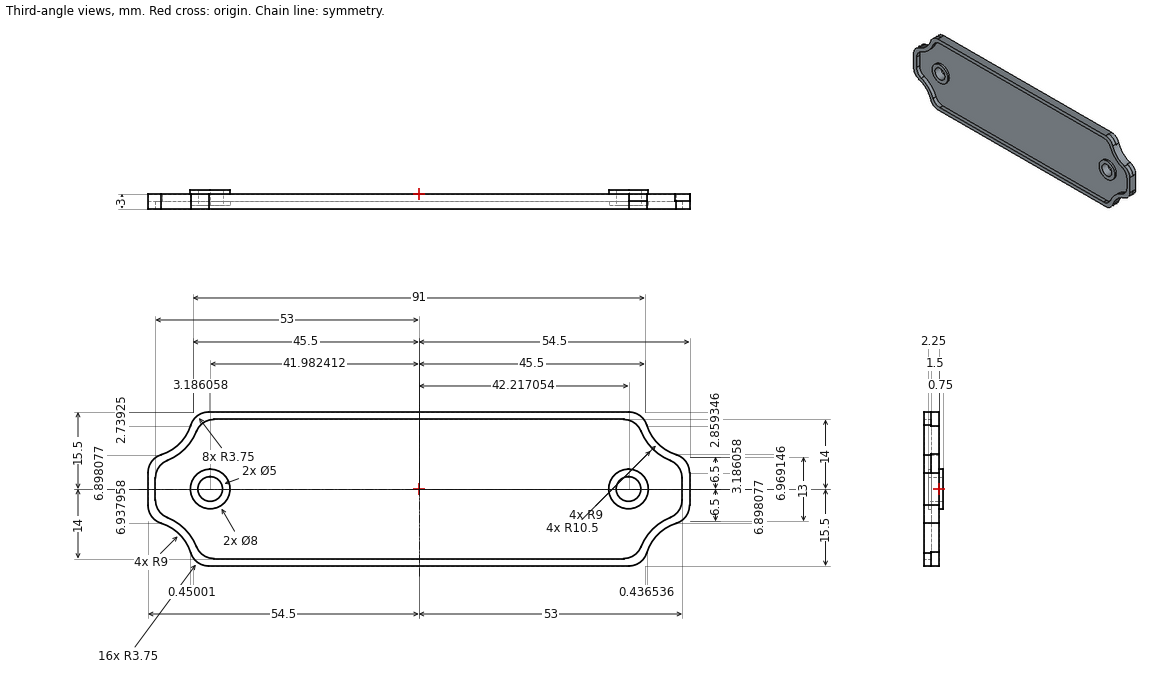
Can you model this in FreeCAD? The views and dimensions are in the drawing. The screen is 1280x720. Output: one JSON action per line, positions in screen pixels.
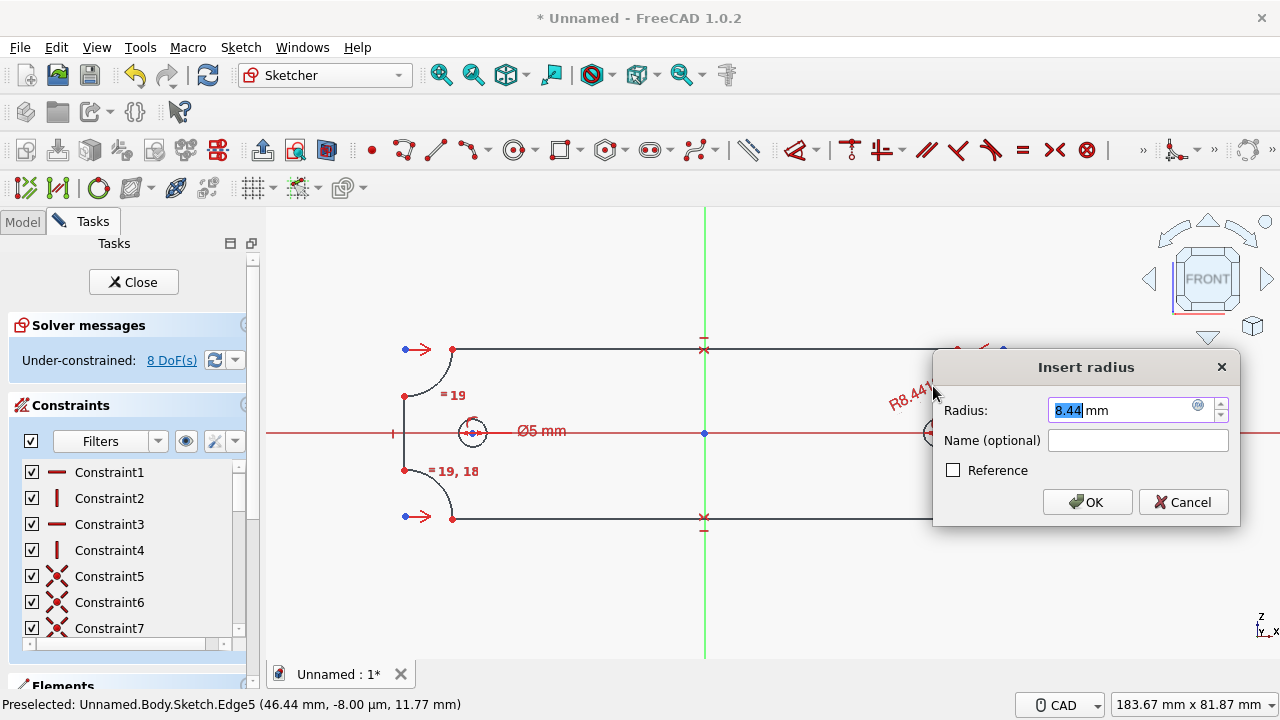
{"action": "type", "text": "9"}
{"action": "key", "text": "Return"}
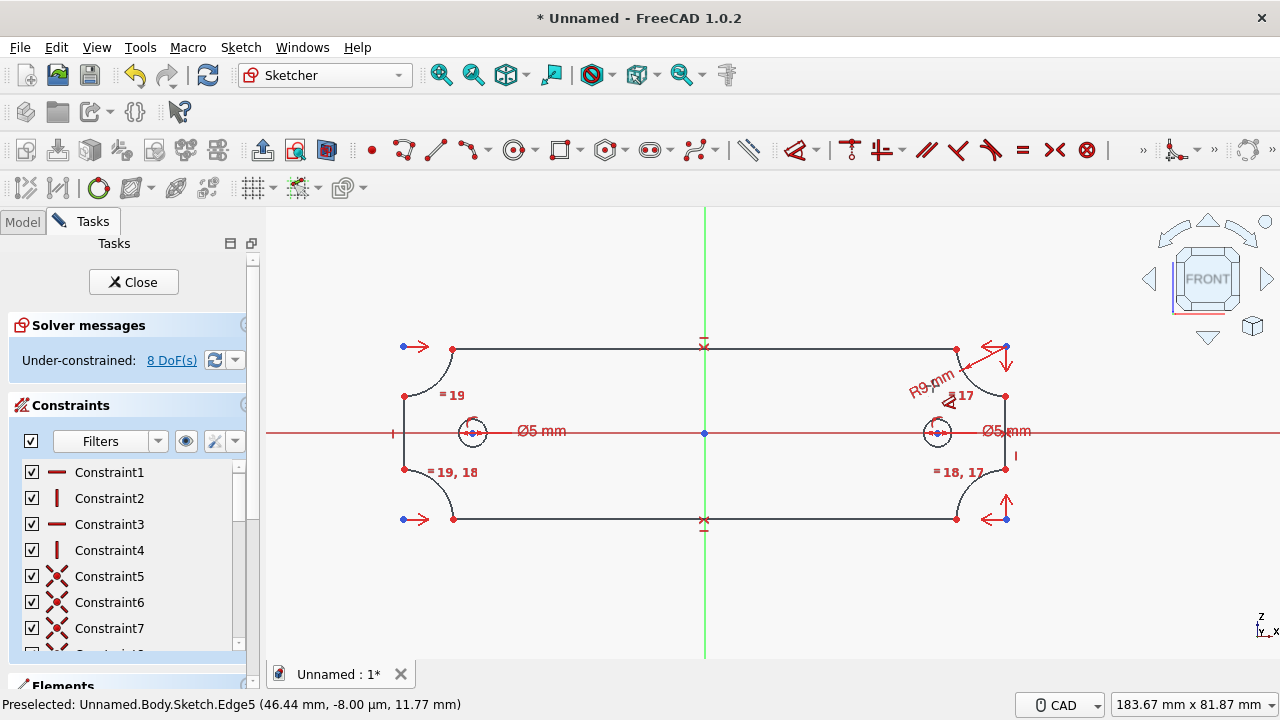
{"action": "left_click", "coordinate": [604, 349]}
{"action": "left_click", "coordinate": [589, 315]}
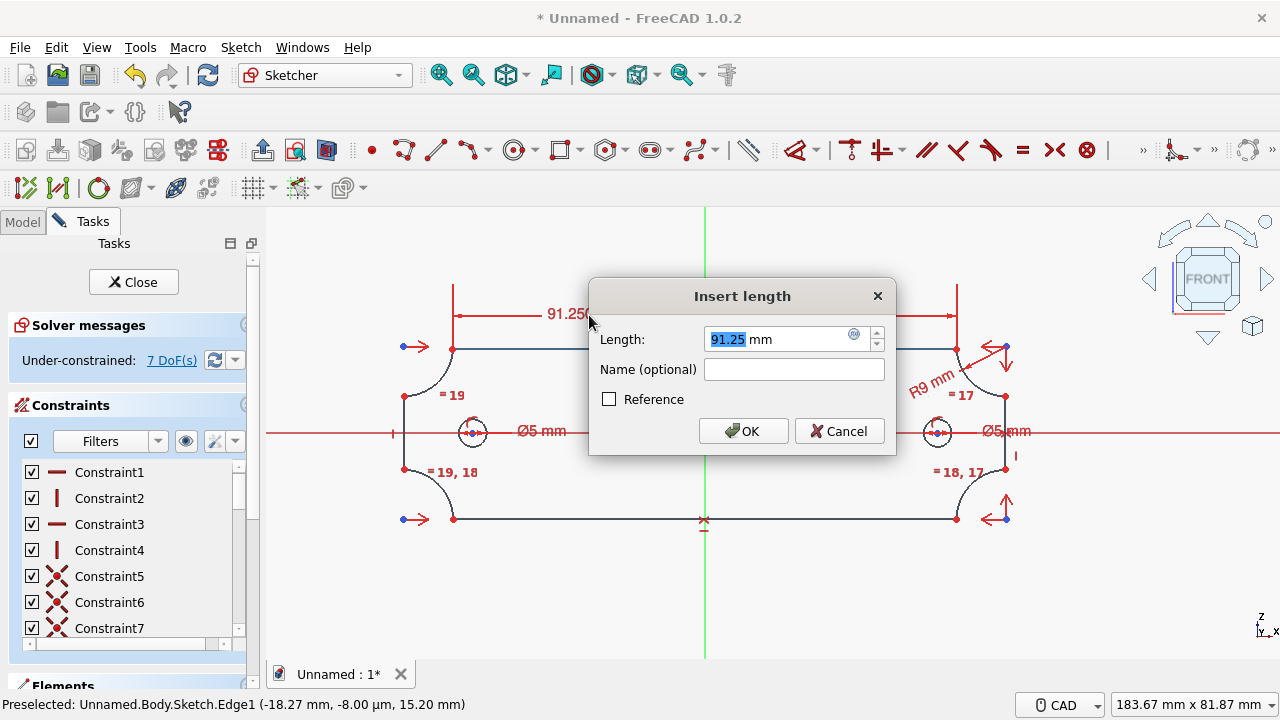
{"action": "type", "text": "91"}
{"action": "key", "text": "Return"}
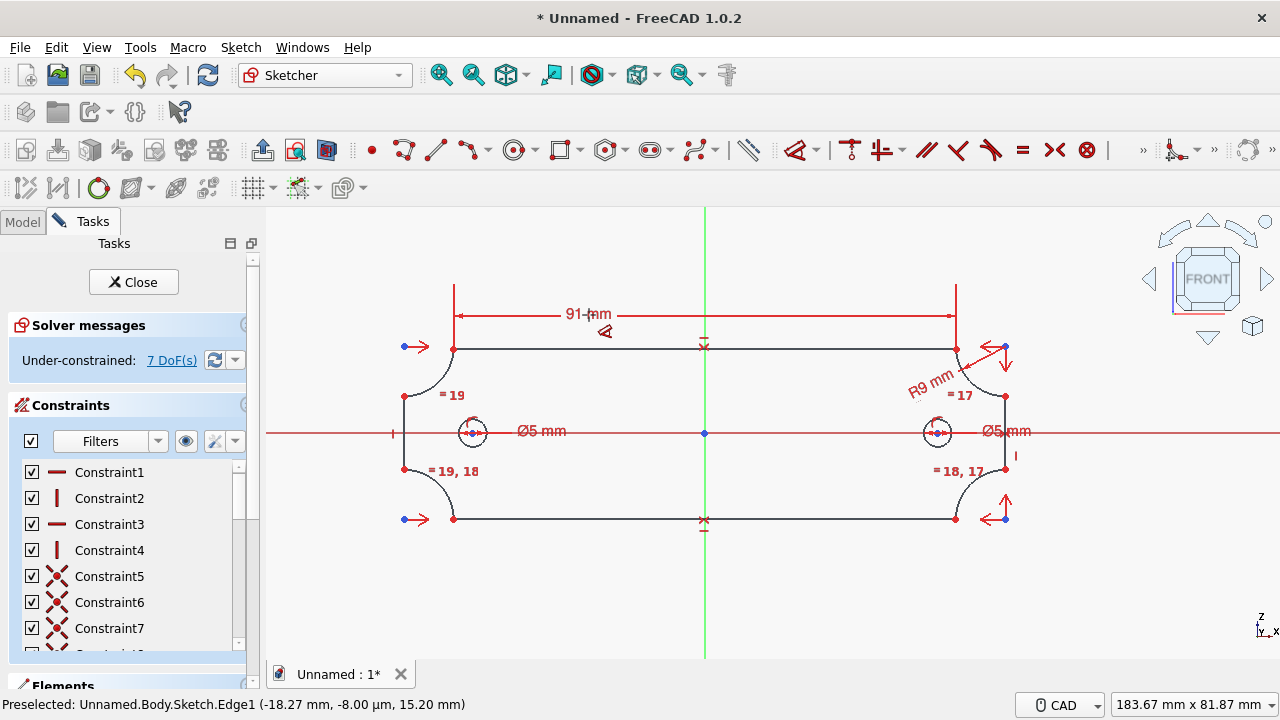
{"action": "left_click", "coordinate": [1005, 418]}
{"action": "left_click", "coordinate": [1039, 416]}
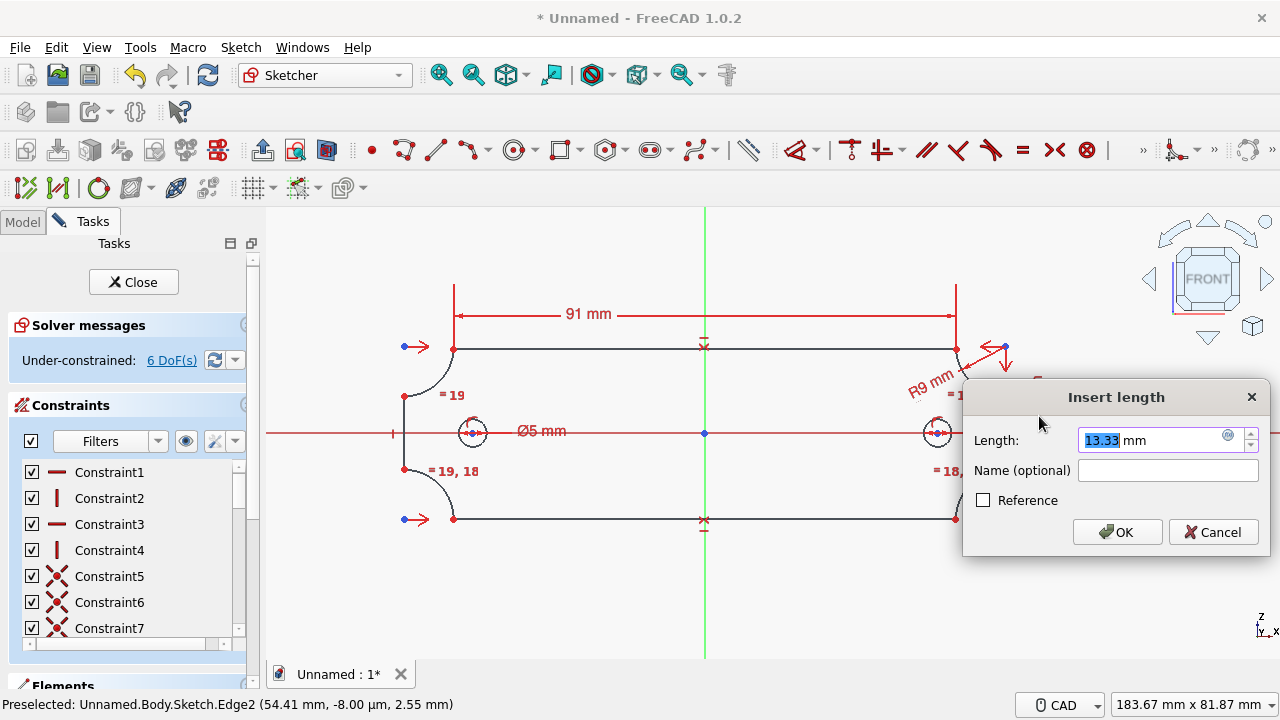
{"action": "type", "text": "13"}
{"action": "key", "text": "Return"}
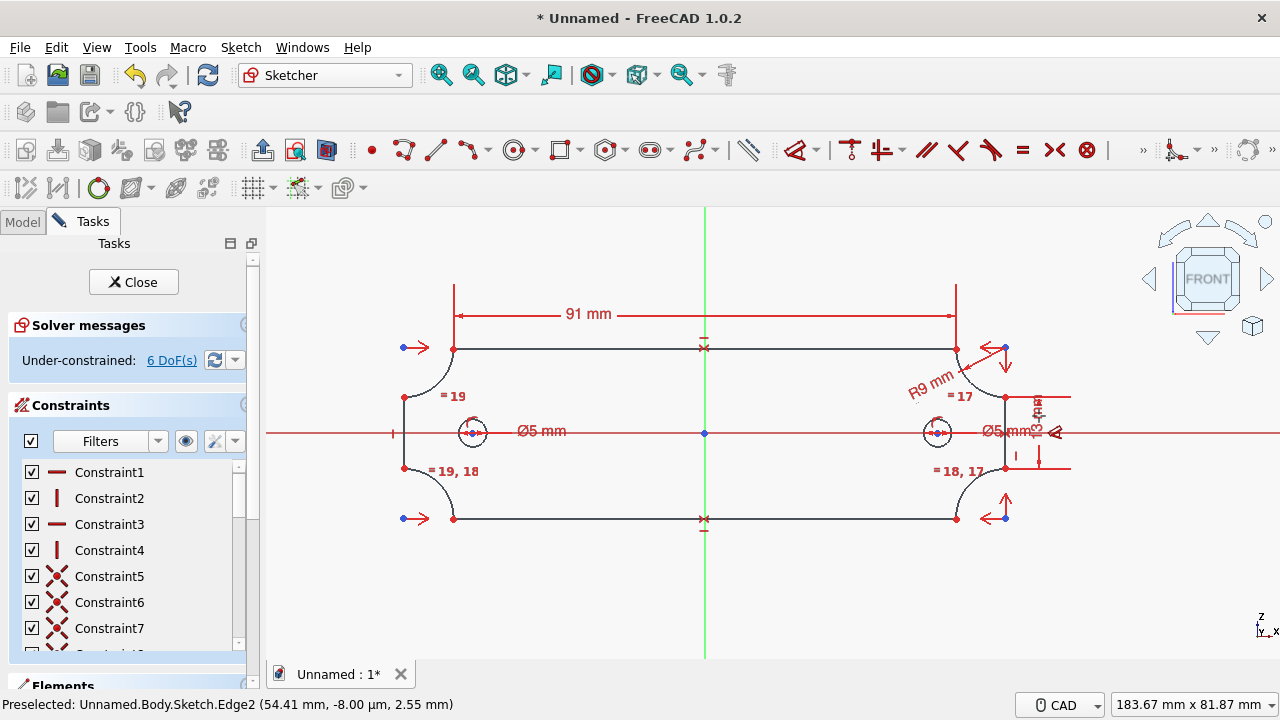
{"action": "left_click", "coordinate": [454, 349]}
{"action": "left_click", "coordinate": [420, 372]}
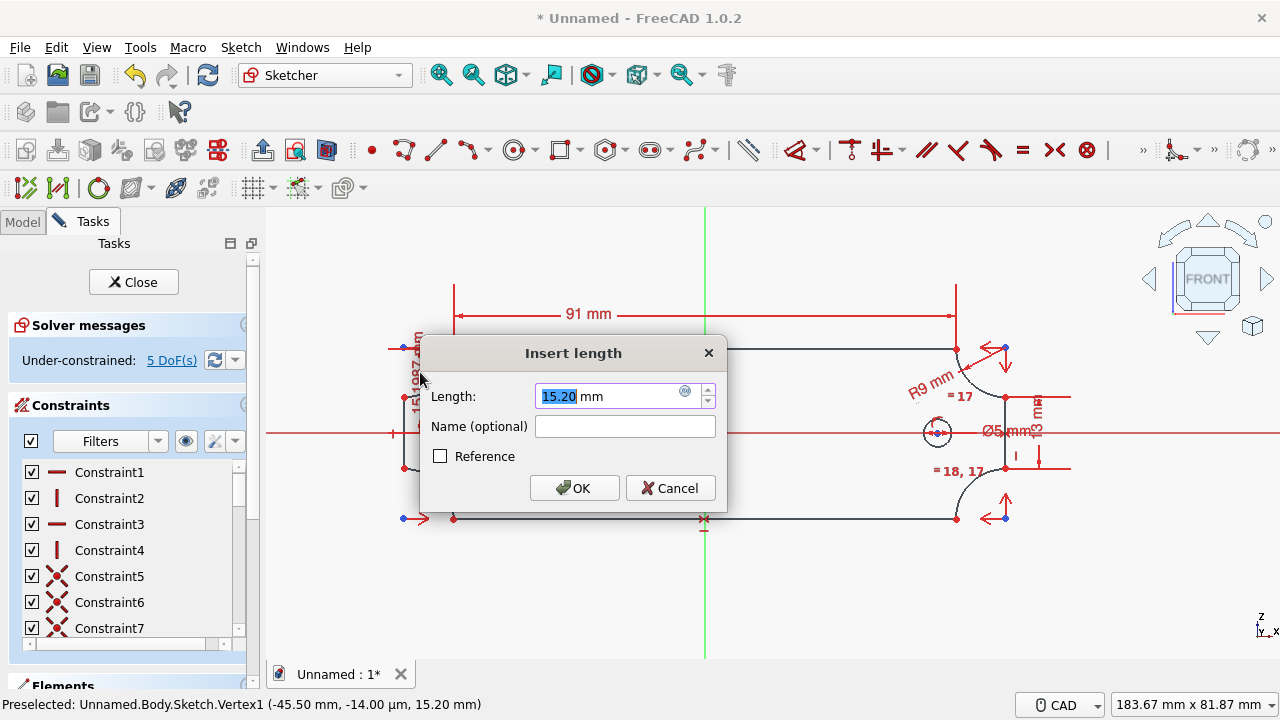
{"action": "type", "text": "15.5"}
{"action": "key", "text": "Return"}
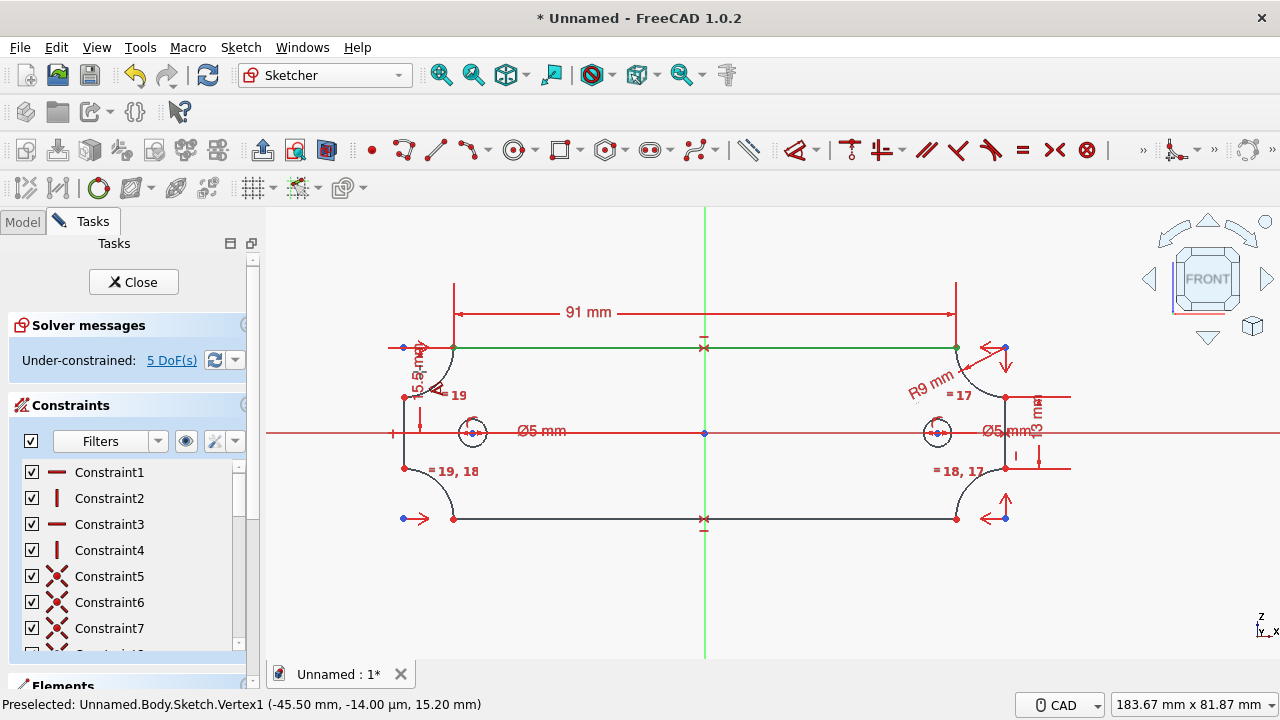
{"action": "left_click", "coordinate": [1005, 397]}
{"action": "left_click", "coordinate": [855, 363]}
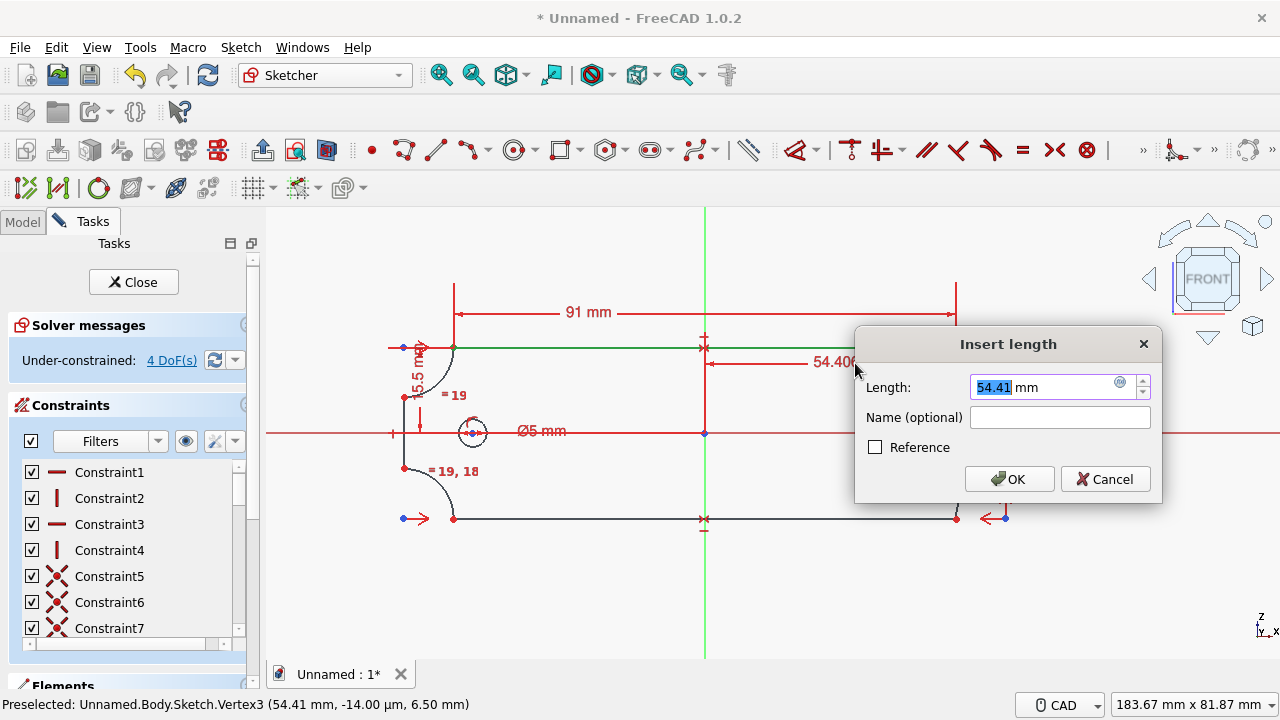
{"action": "type", "text": "54.5"}
{"action": "key", "text": "Return"}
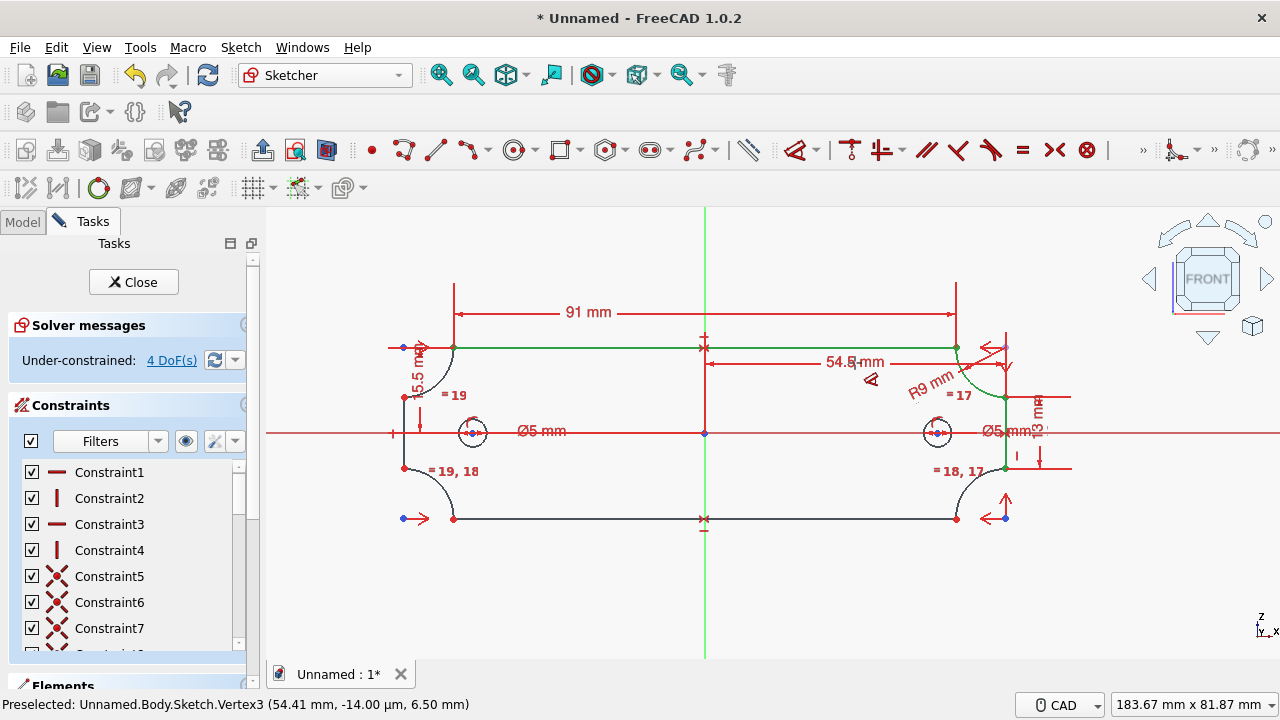
{"action": "left_click", "coordinate": [956, 519]}
{"action": "left_click", "coordinate": [990, 456]}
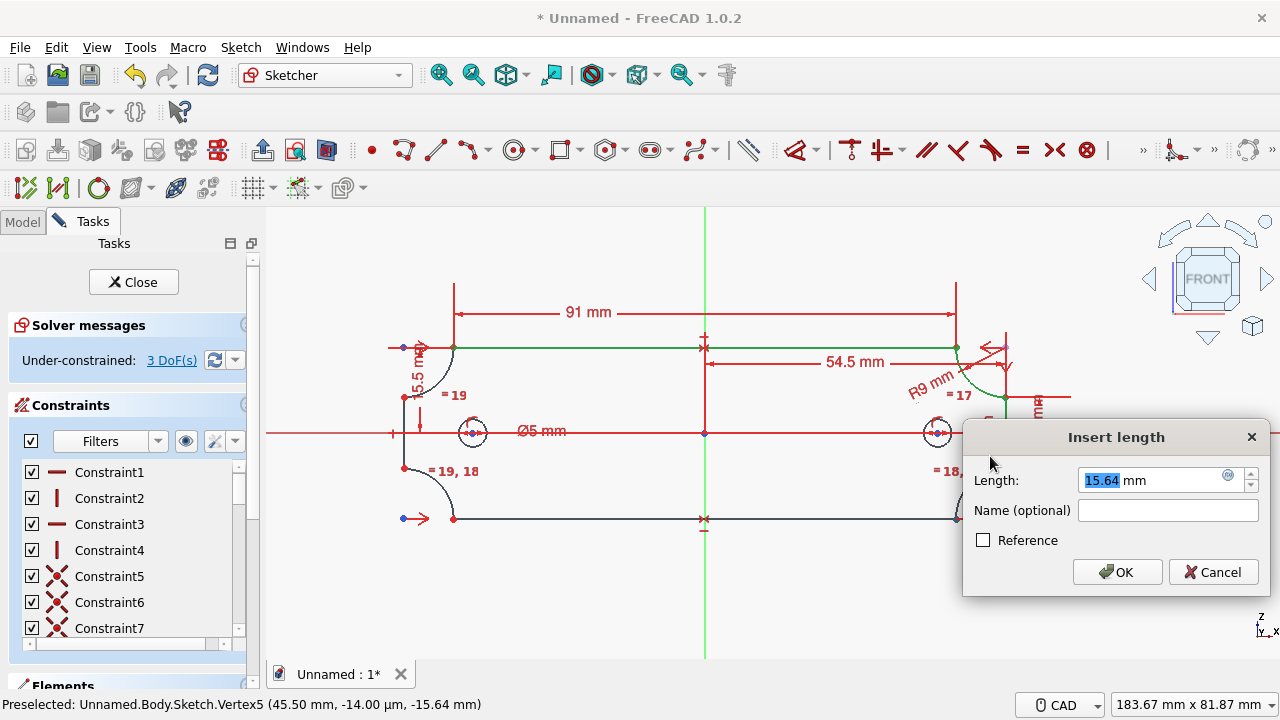
{"action": "type", "text": "15.5"}
{"action": "key", "text": "Return"}